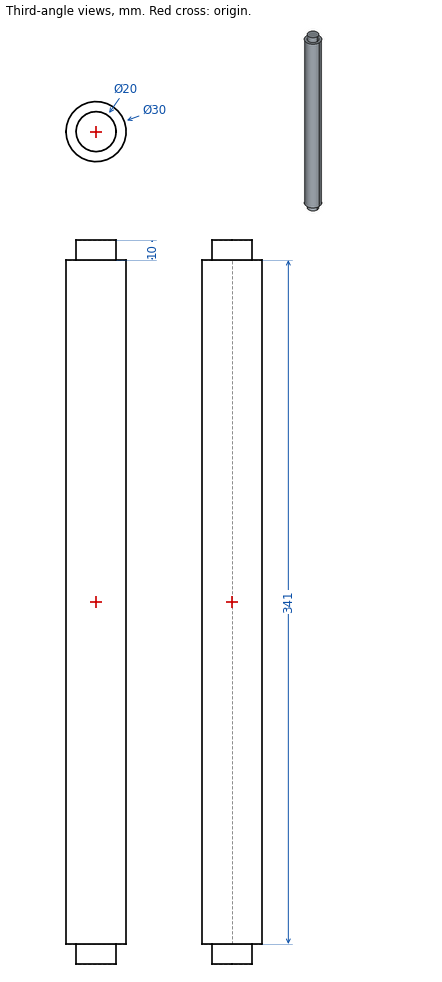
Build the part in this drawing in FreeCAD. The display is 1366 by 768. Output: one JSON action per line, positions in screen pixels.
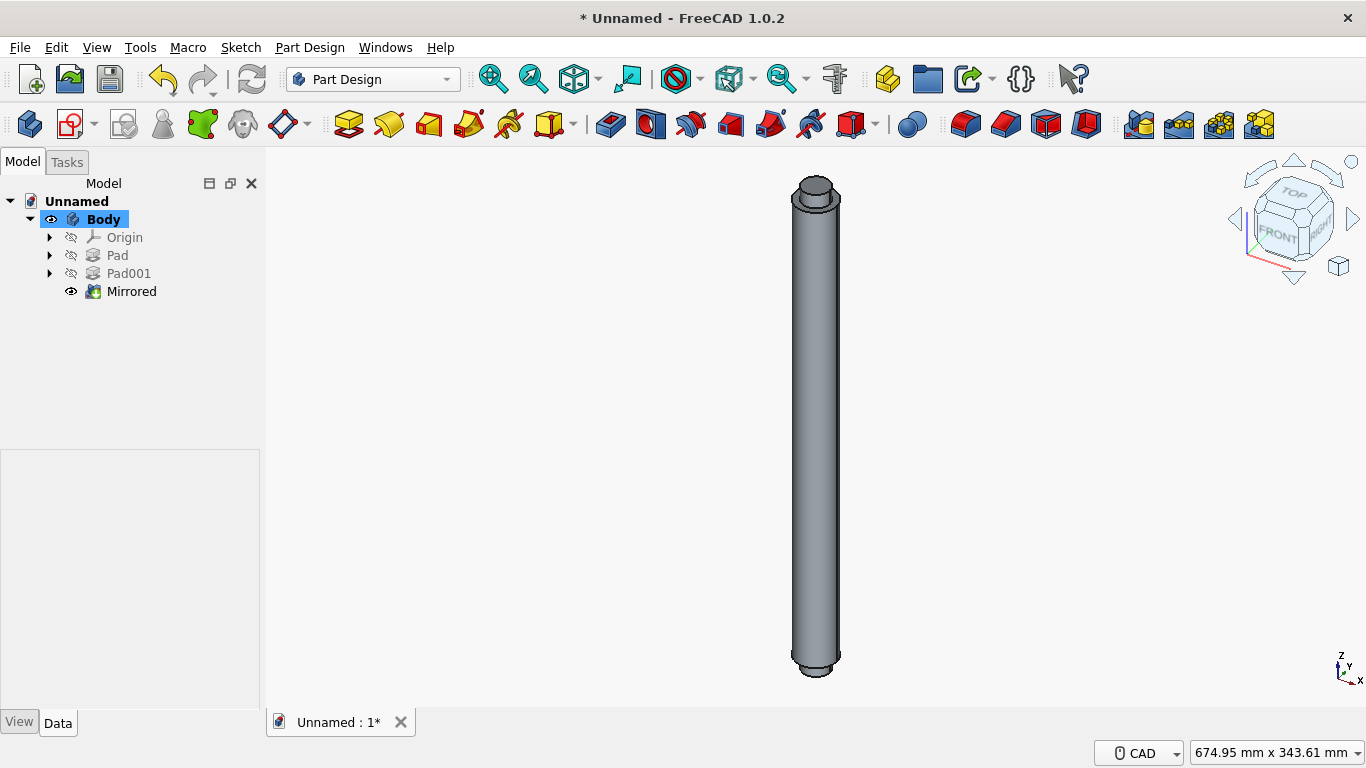
{"action": "key", "text": "0"}